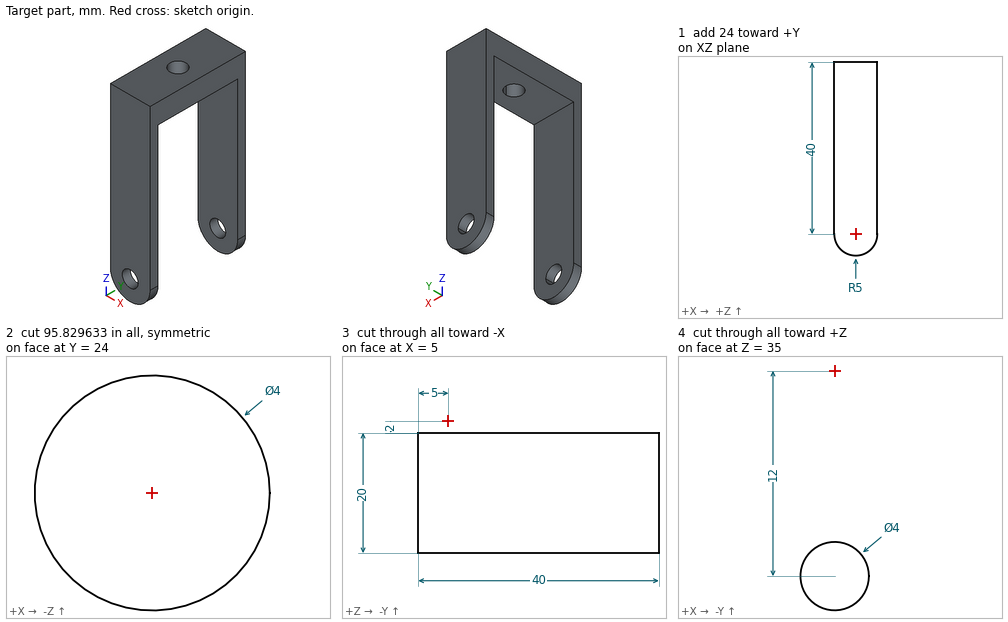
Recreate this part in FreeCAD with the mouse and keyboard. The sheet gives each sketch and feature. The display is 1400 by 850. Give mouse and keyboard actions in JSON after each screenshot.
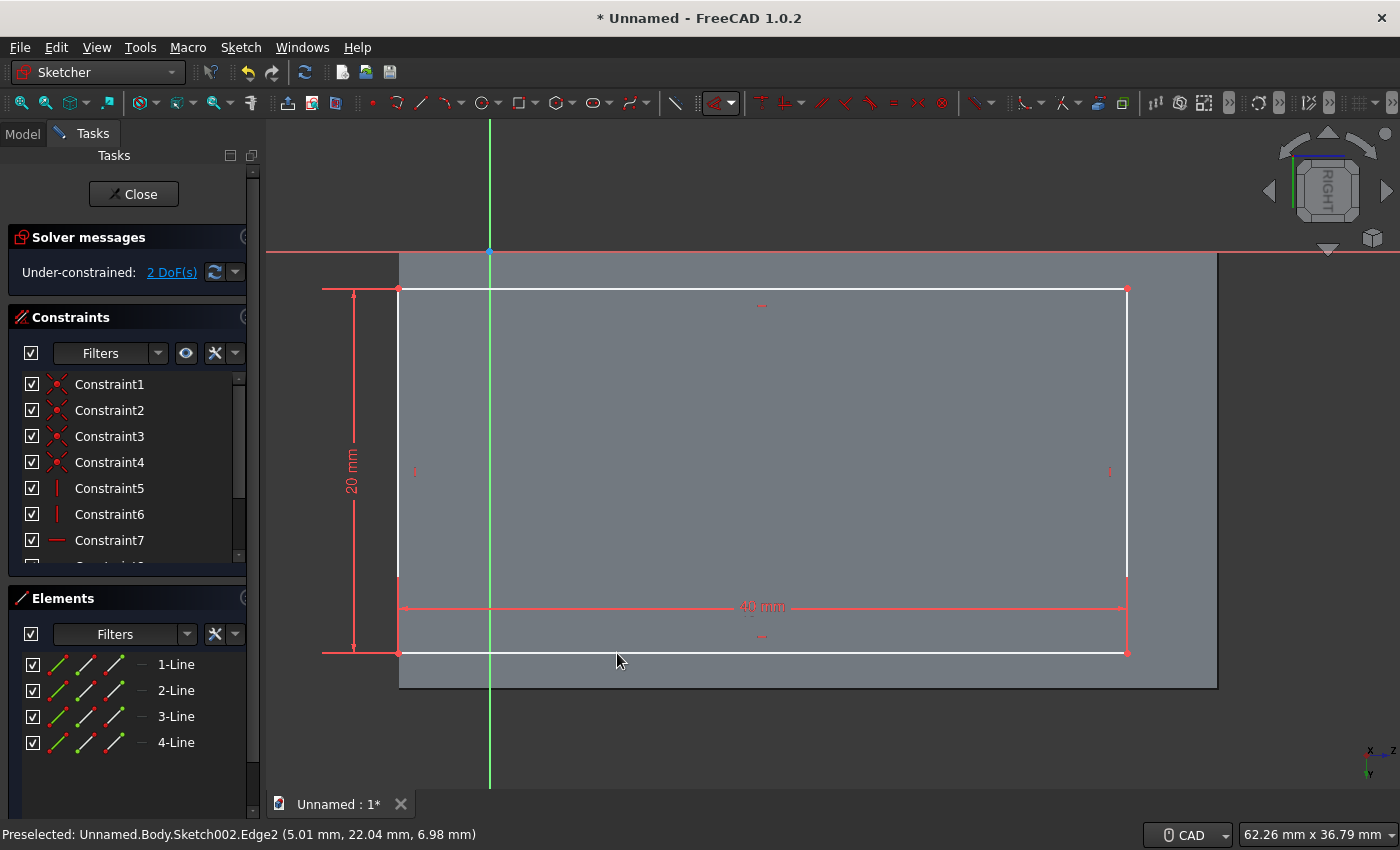
{"action": "left_click", "coordinate": [399, 289]}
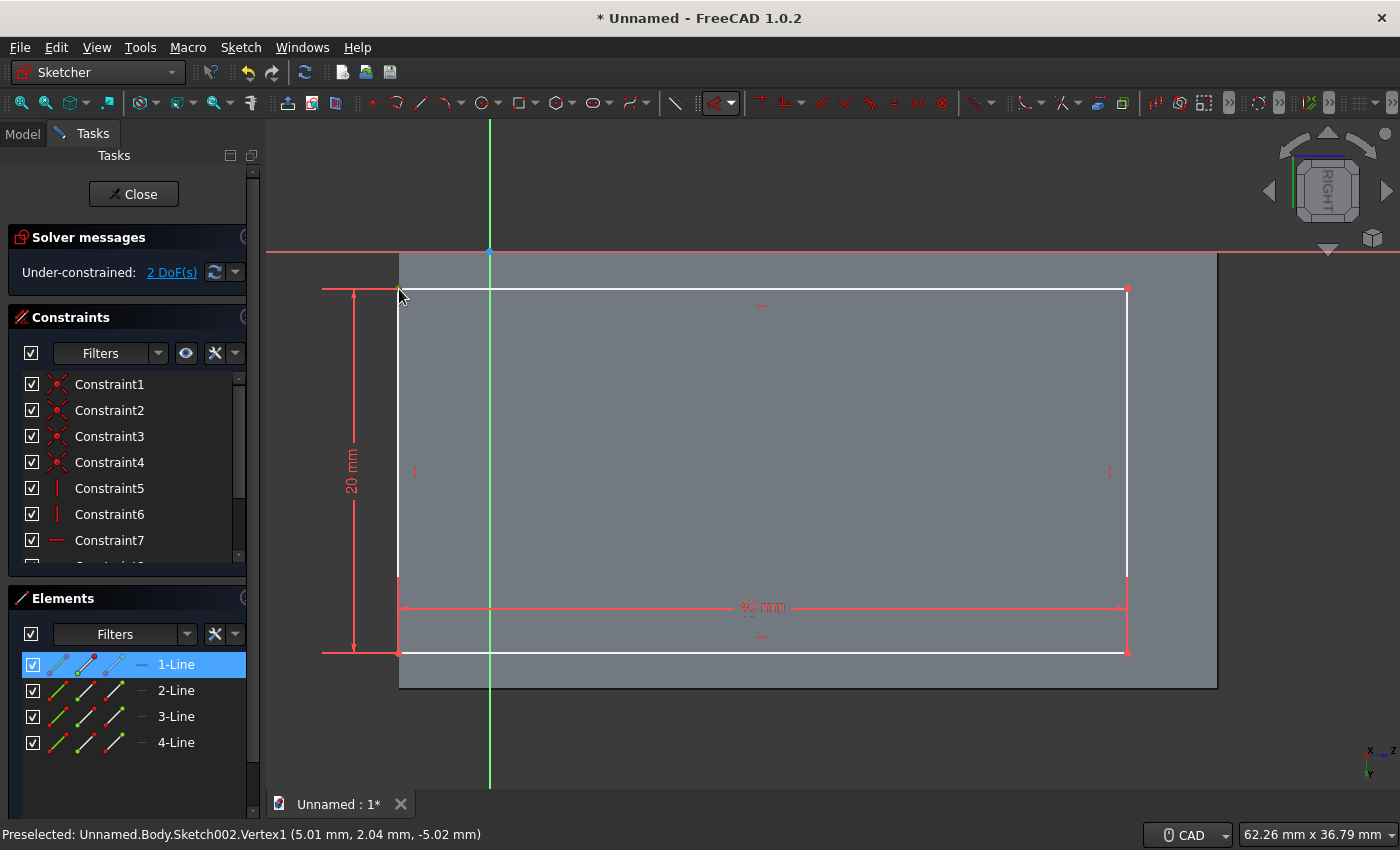
{"action": "key", "text": "l"}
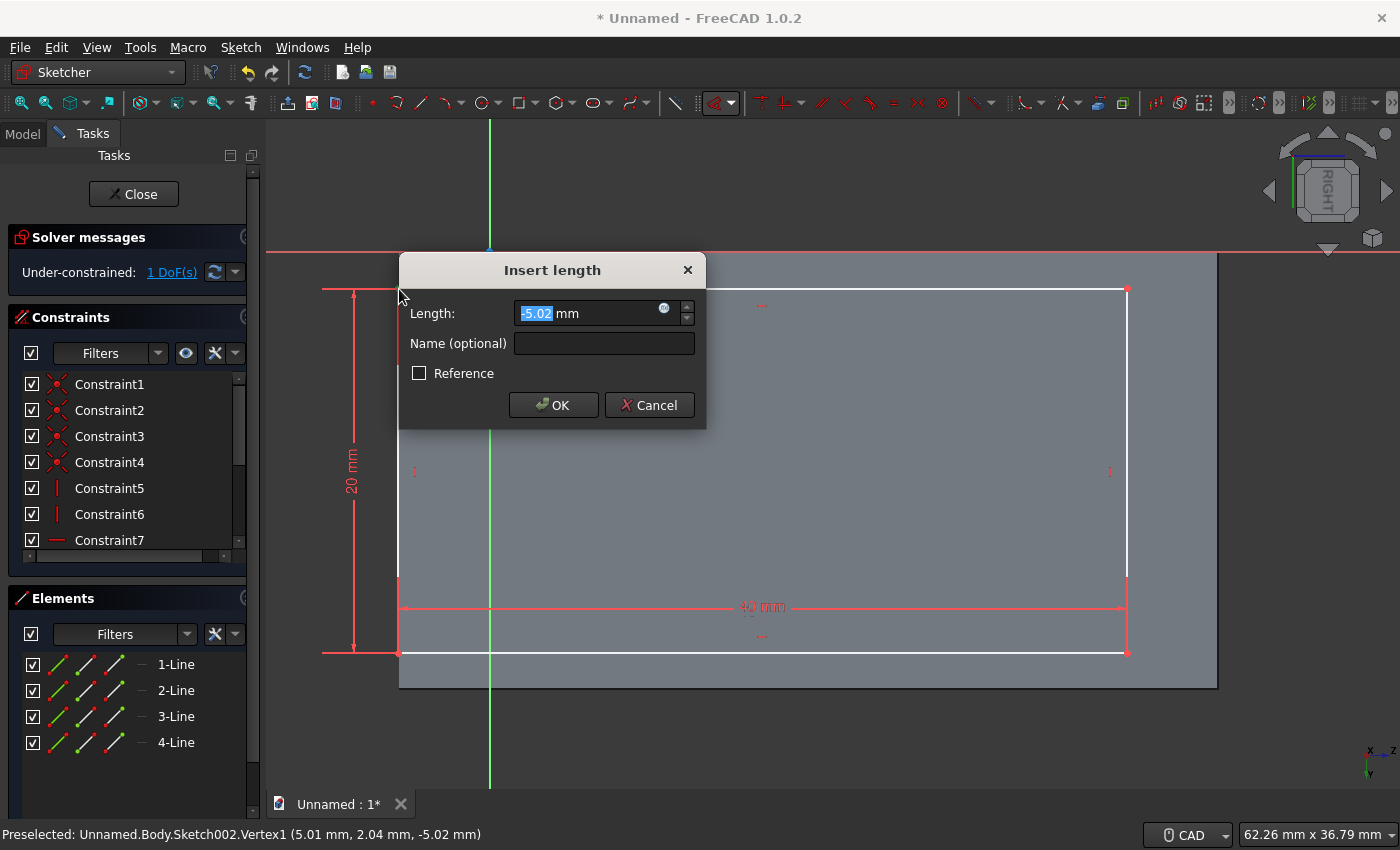
{"action": "type", "text": "-5"}
{"action": "key", "text": "Return"}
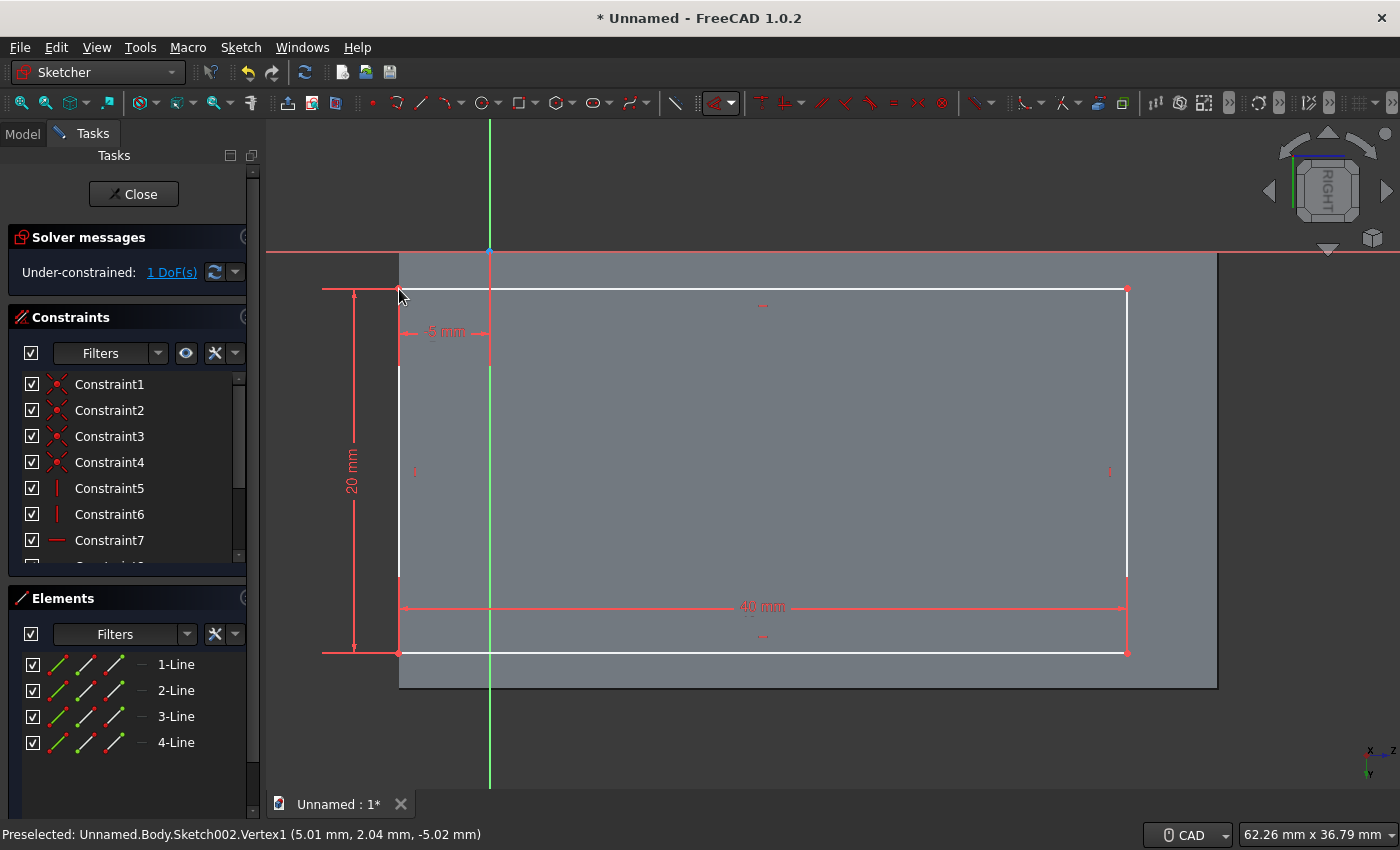
{"action": "left_click", "coordinate": [399, 289]}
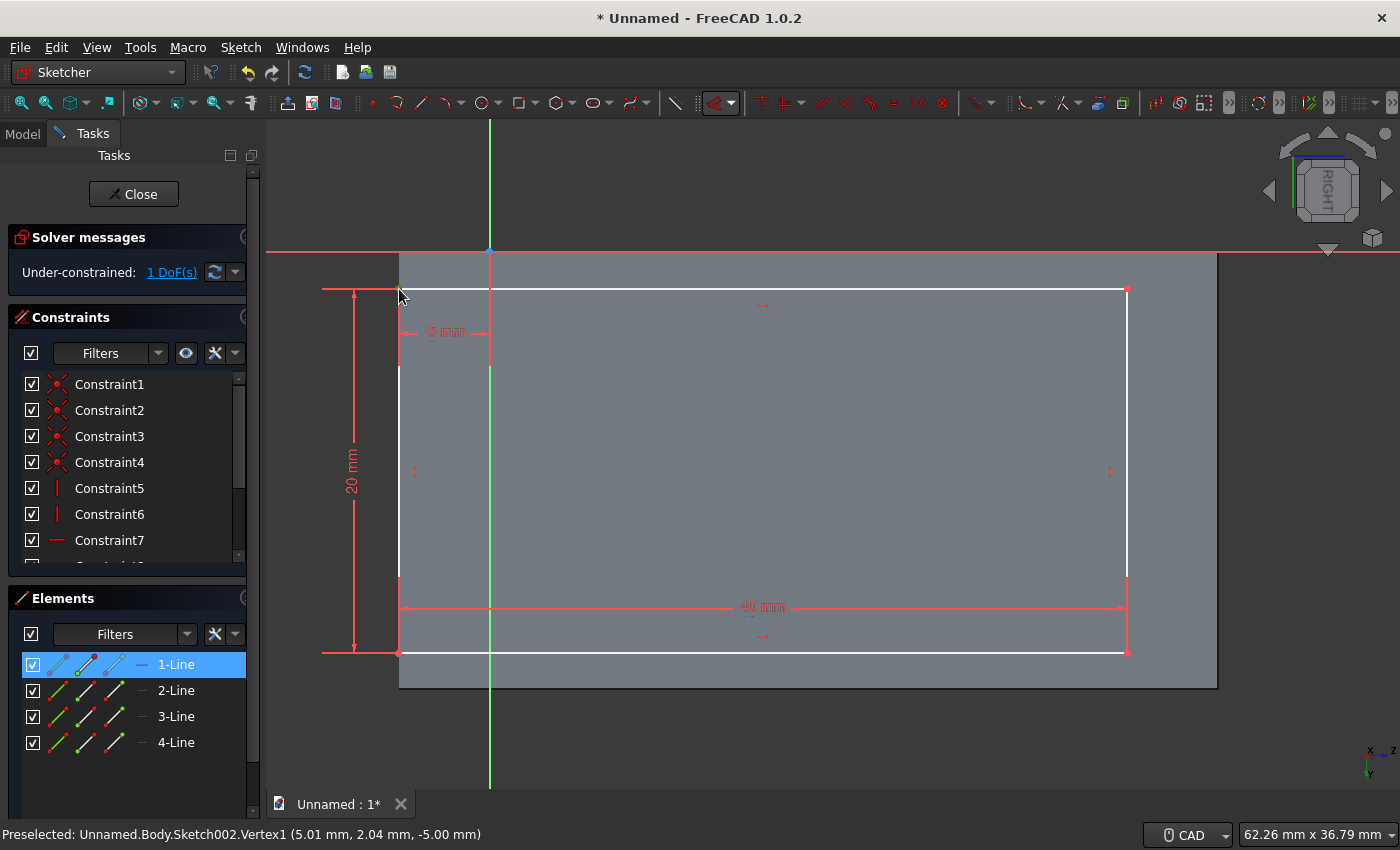
{"action": "key", "text": "i"}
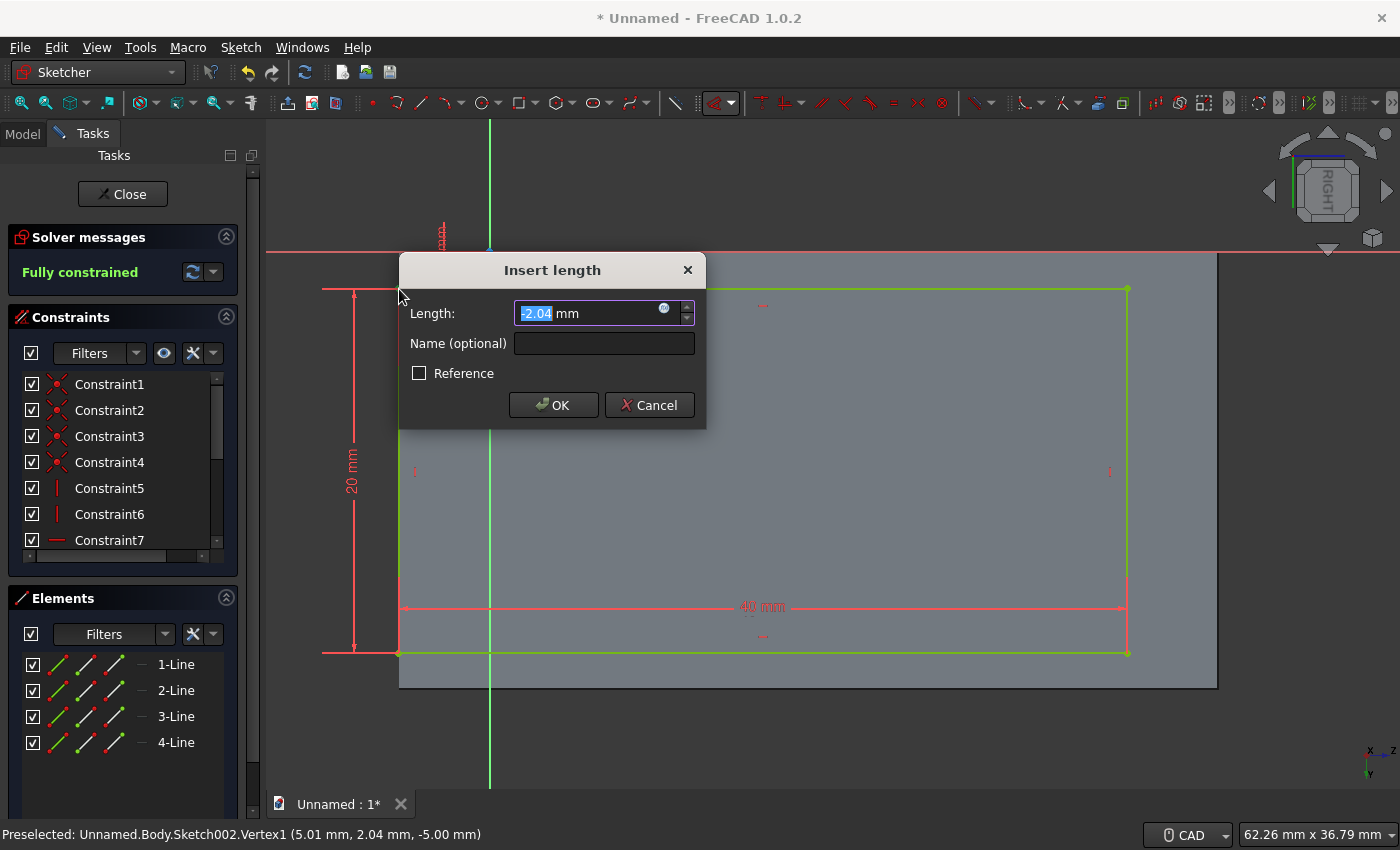
{"action": "type", "text": "-2"}
{"action": "key", "text": "Return"}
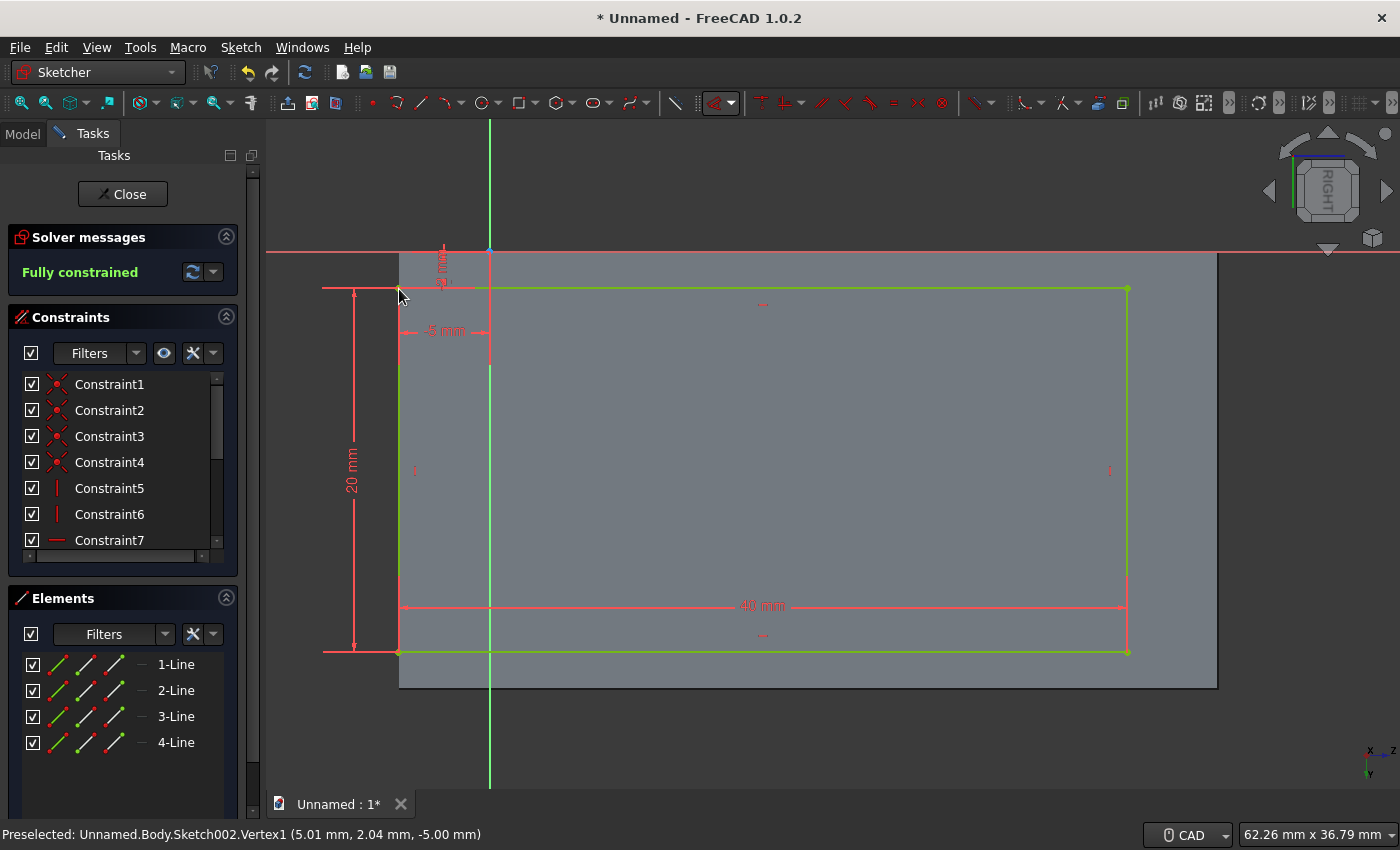
{"action": "left_click", "coordinate": [123, 194]}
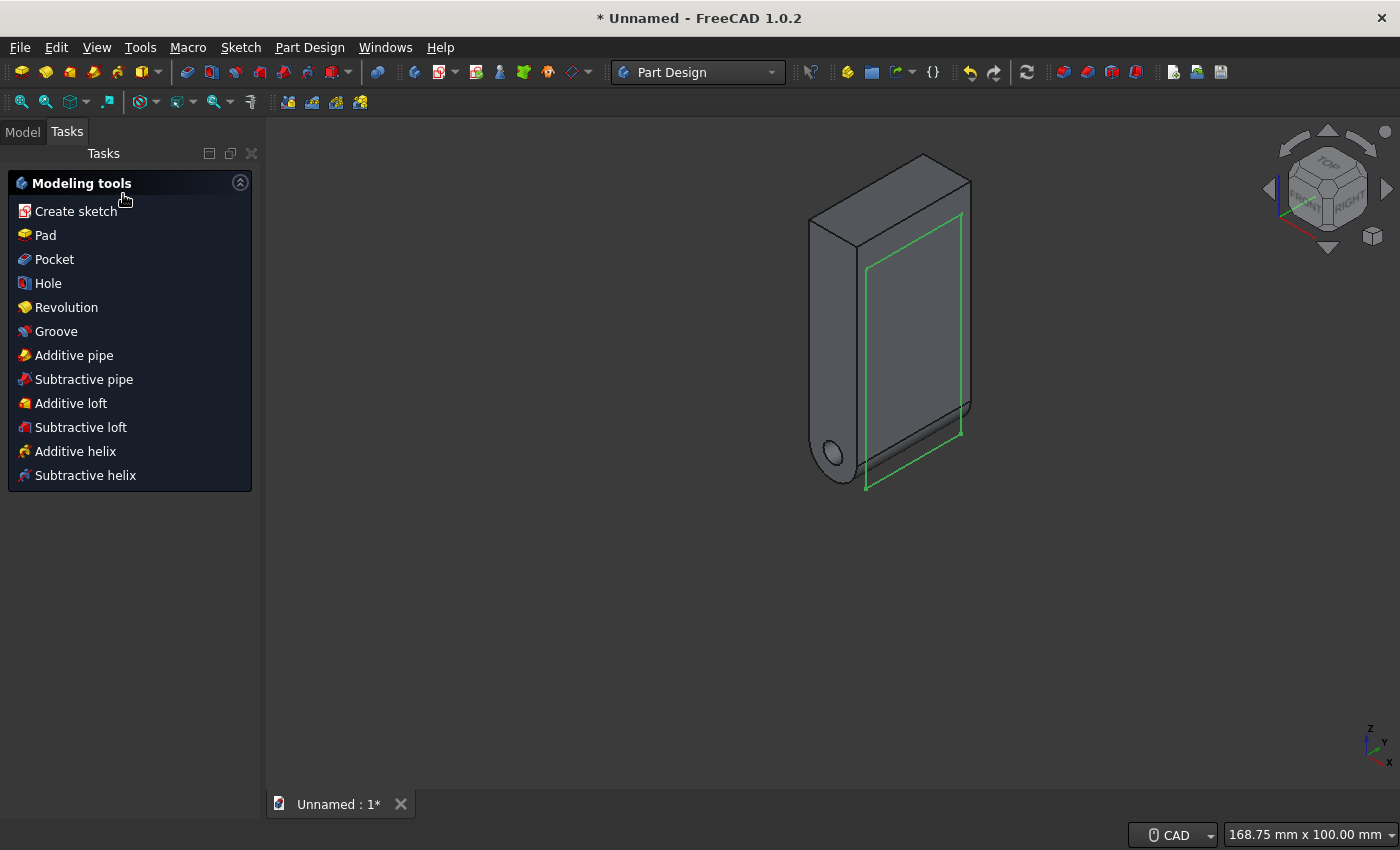
{"action": "left_click", "coordinate": [188, 72]}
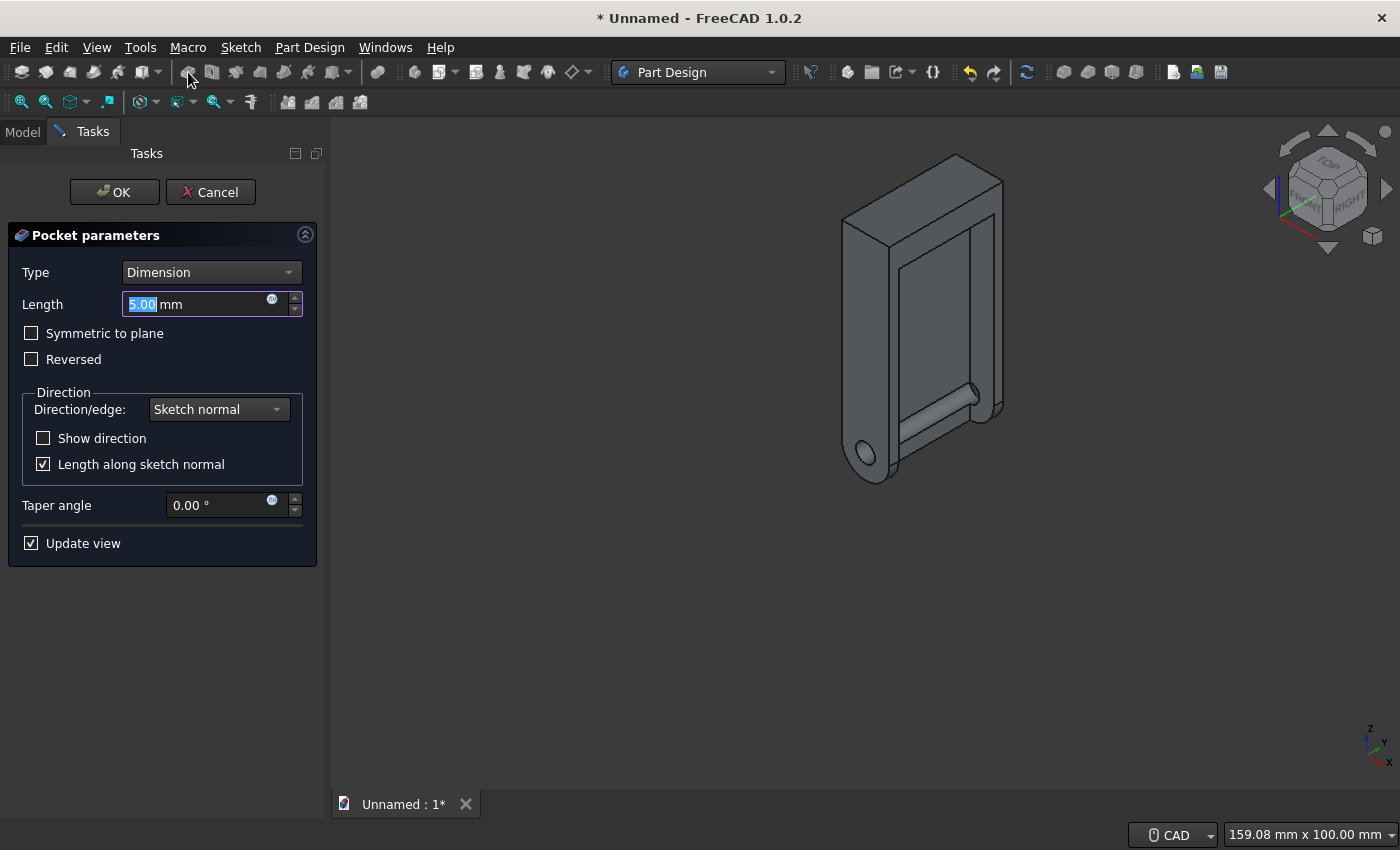
{"action": "left_click", "coordinate": [212, 272]}